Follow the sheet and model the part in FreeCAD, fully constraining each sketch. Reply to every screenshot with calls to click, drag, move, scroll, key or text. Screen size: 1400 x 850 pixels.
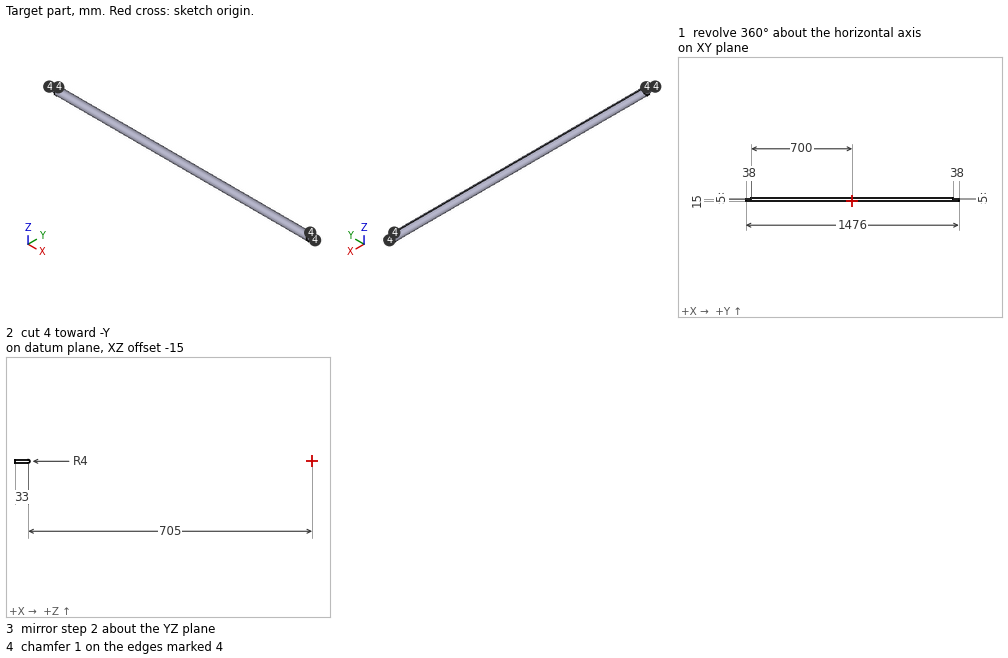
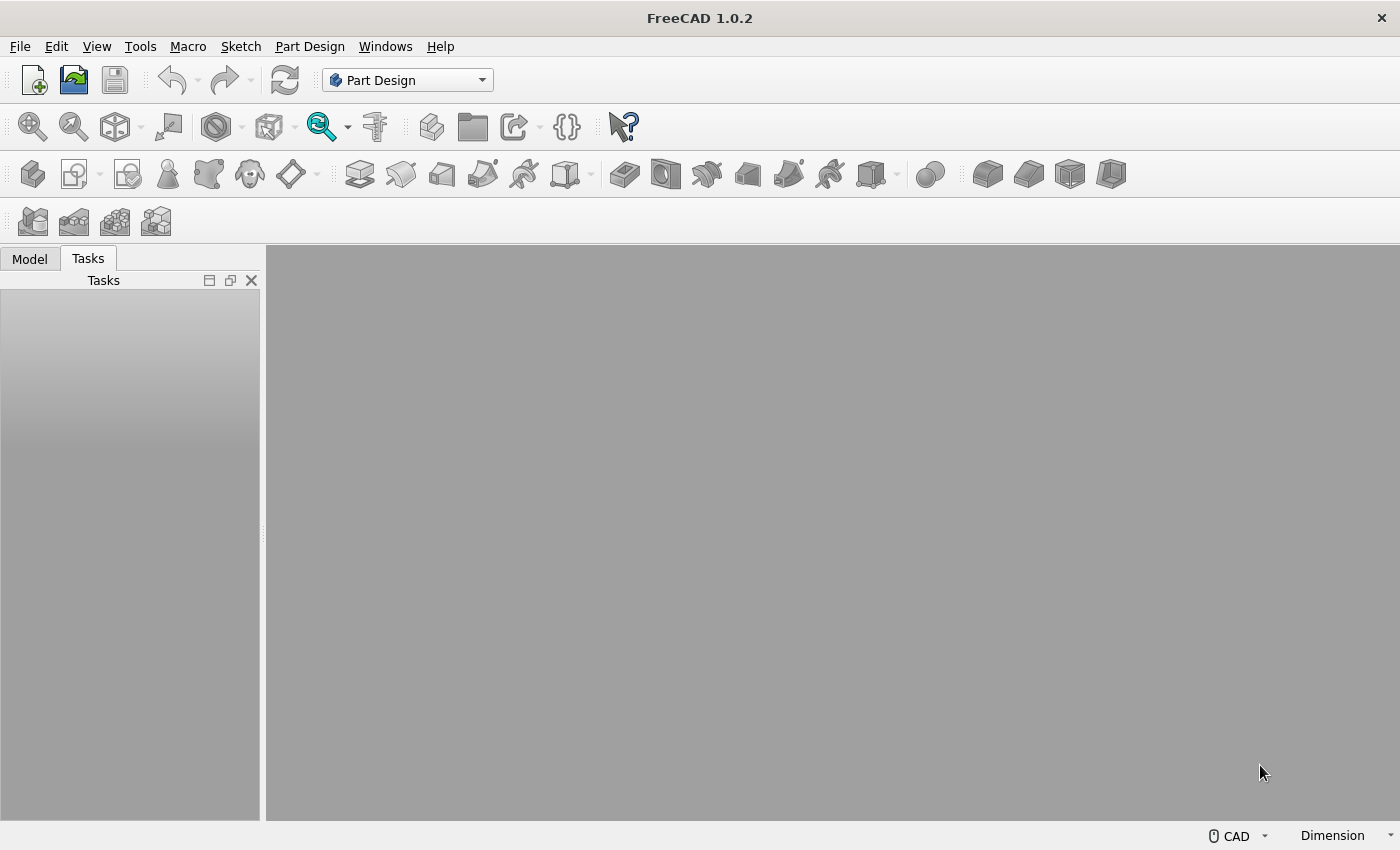
click(33, 80)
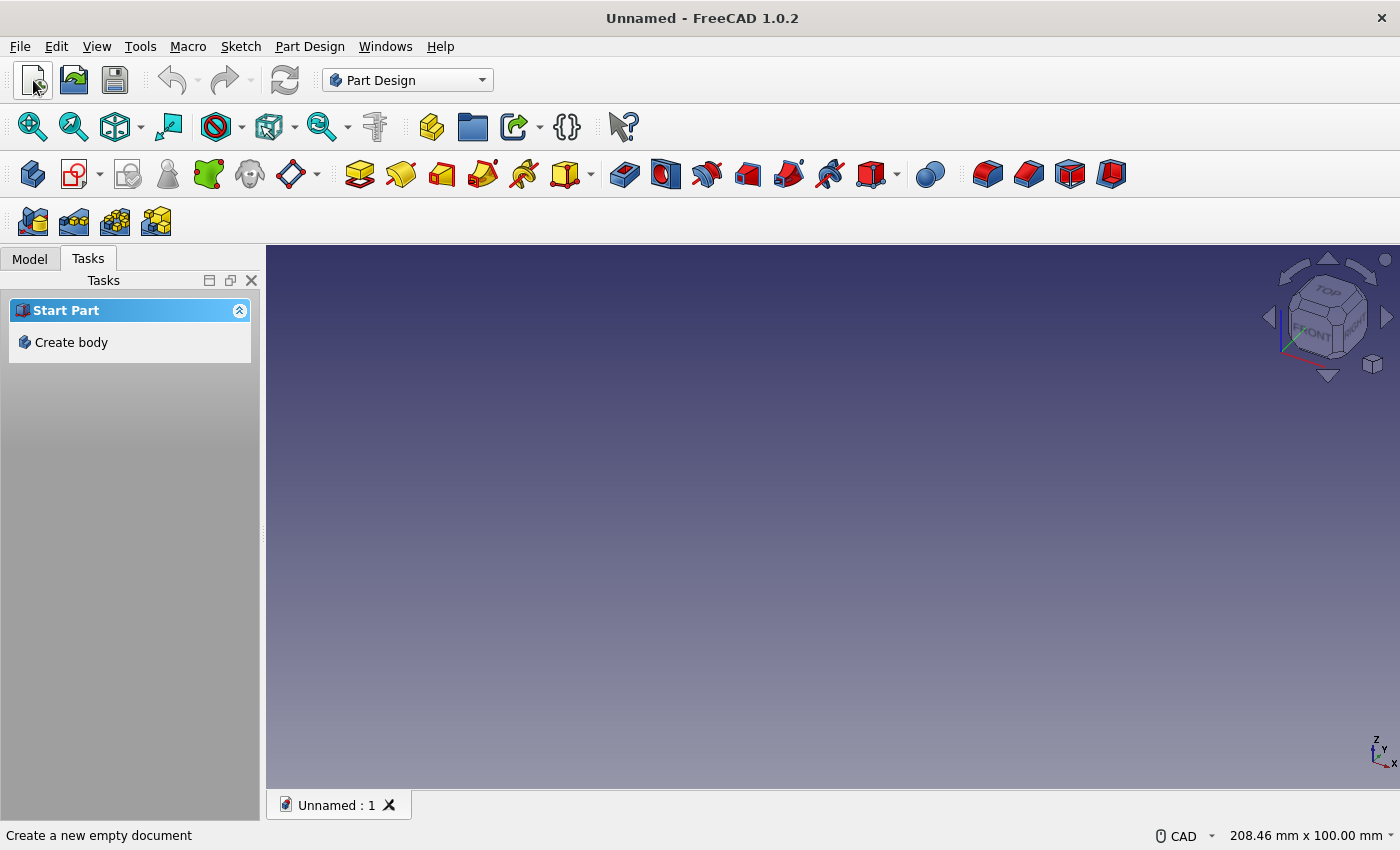
click(74, 174)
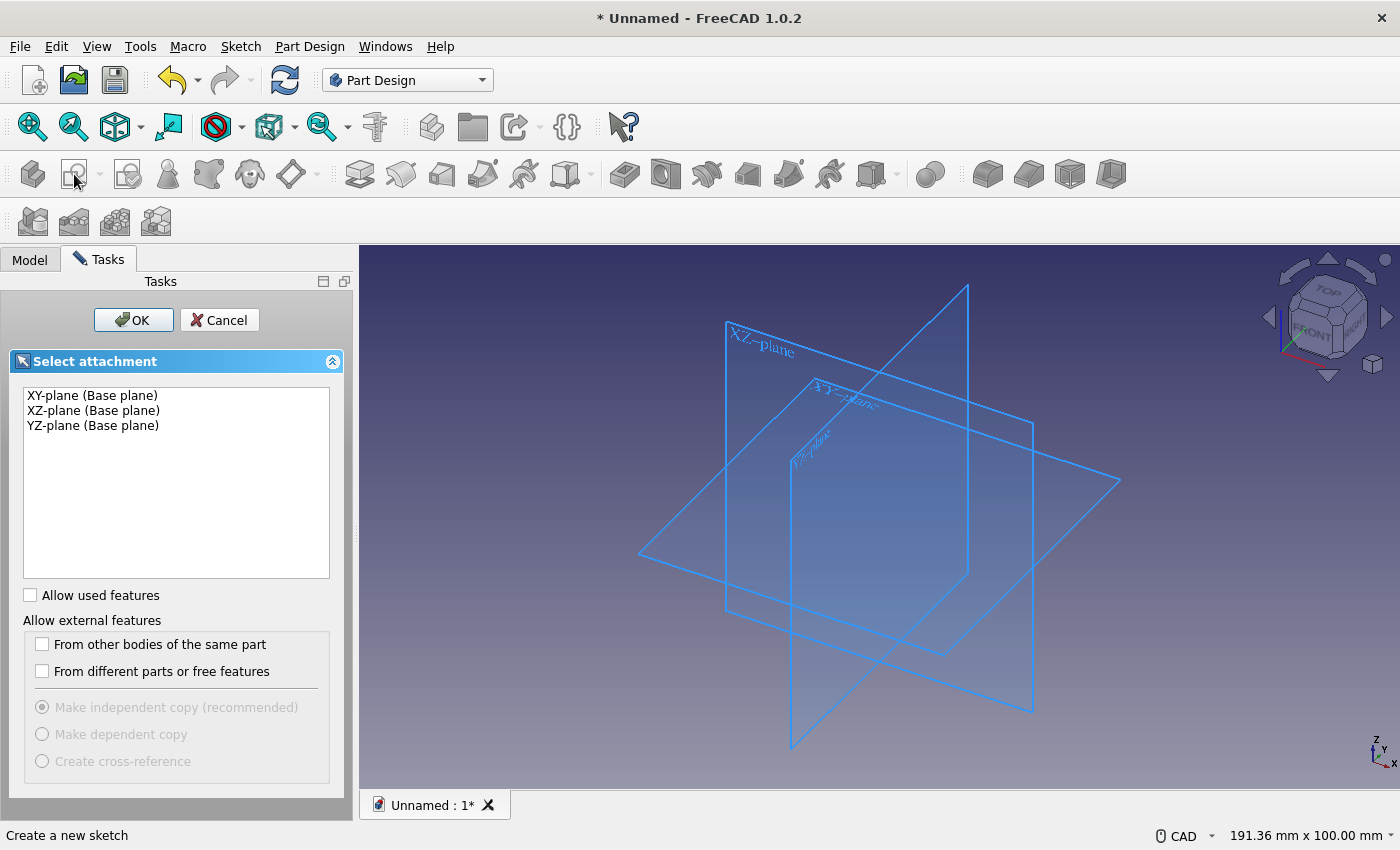
click(84, 396)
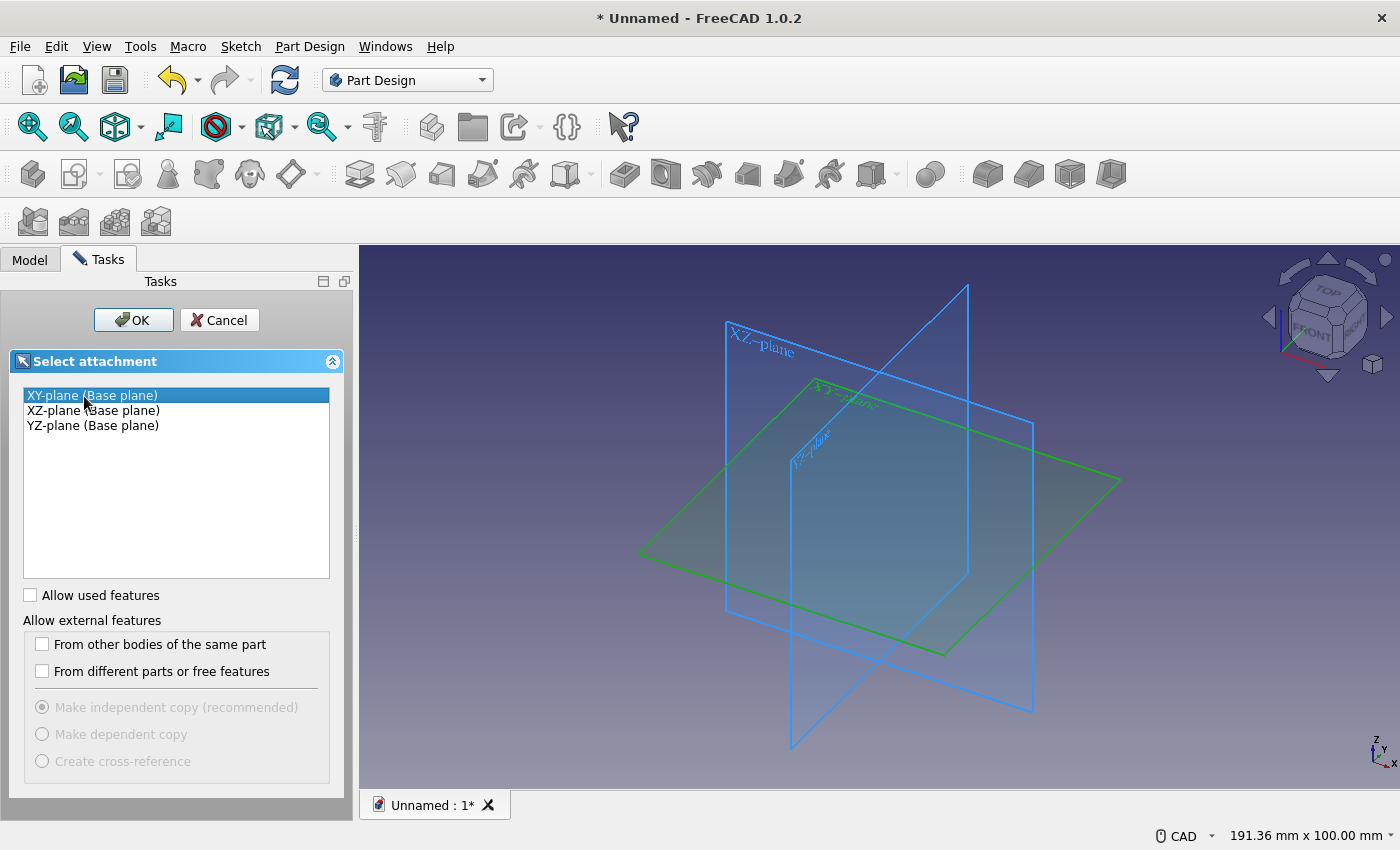
click(134, 320)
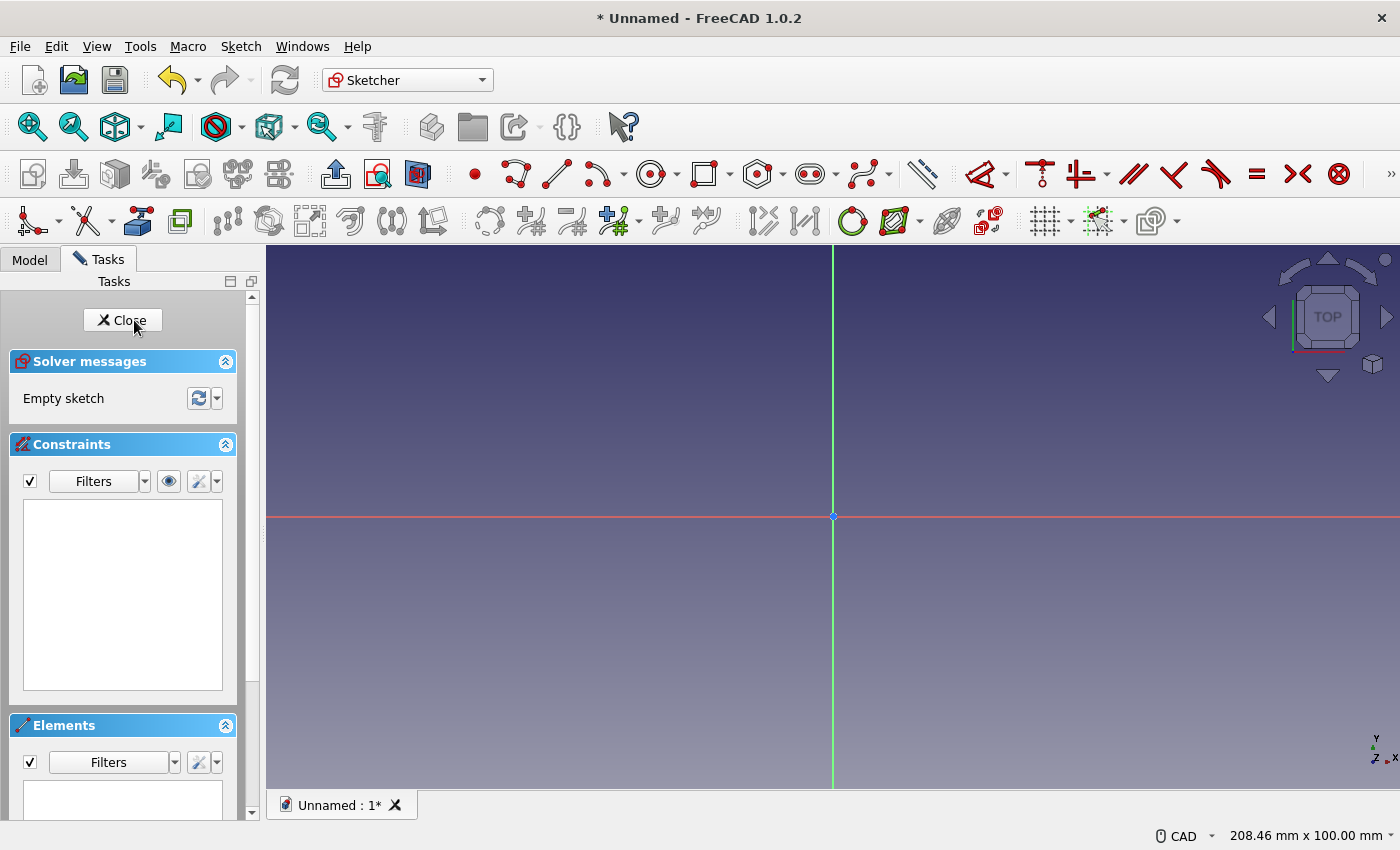
scroll(758, 522, down, 12)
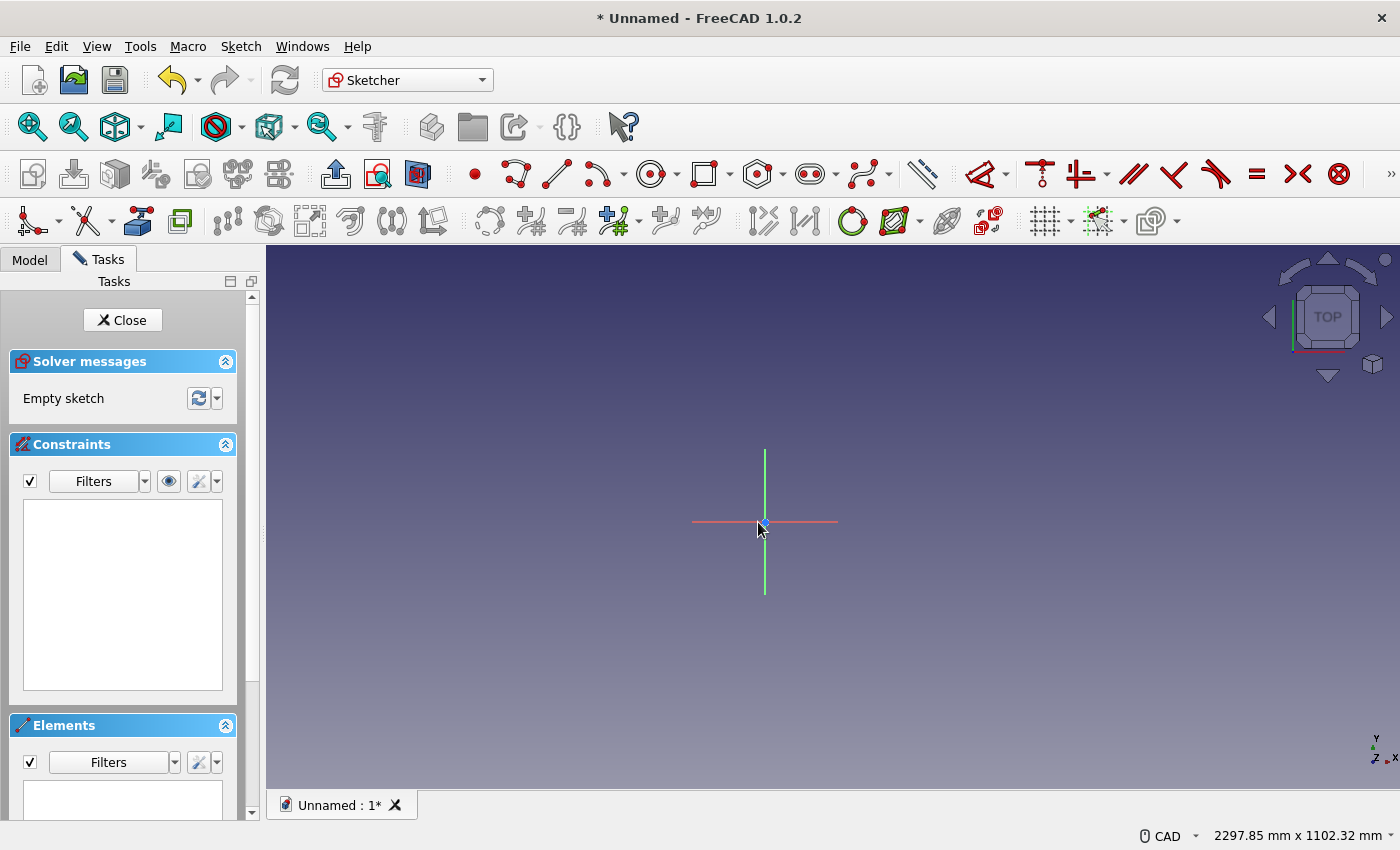
click(516, 174)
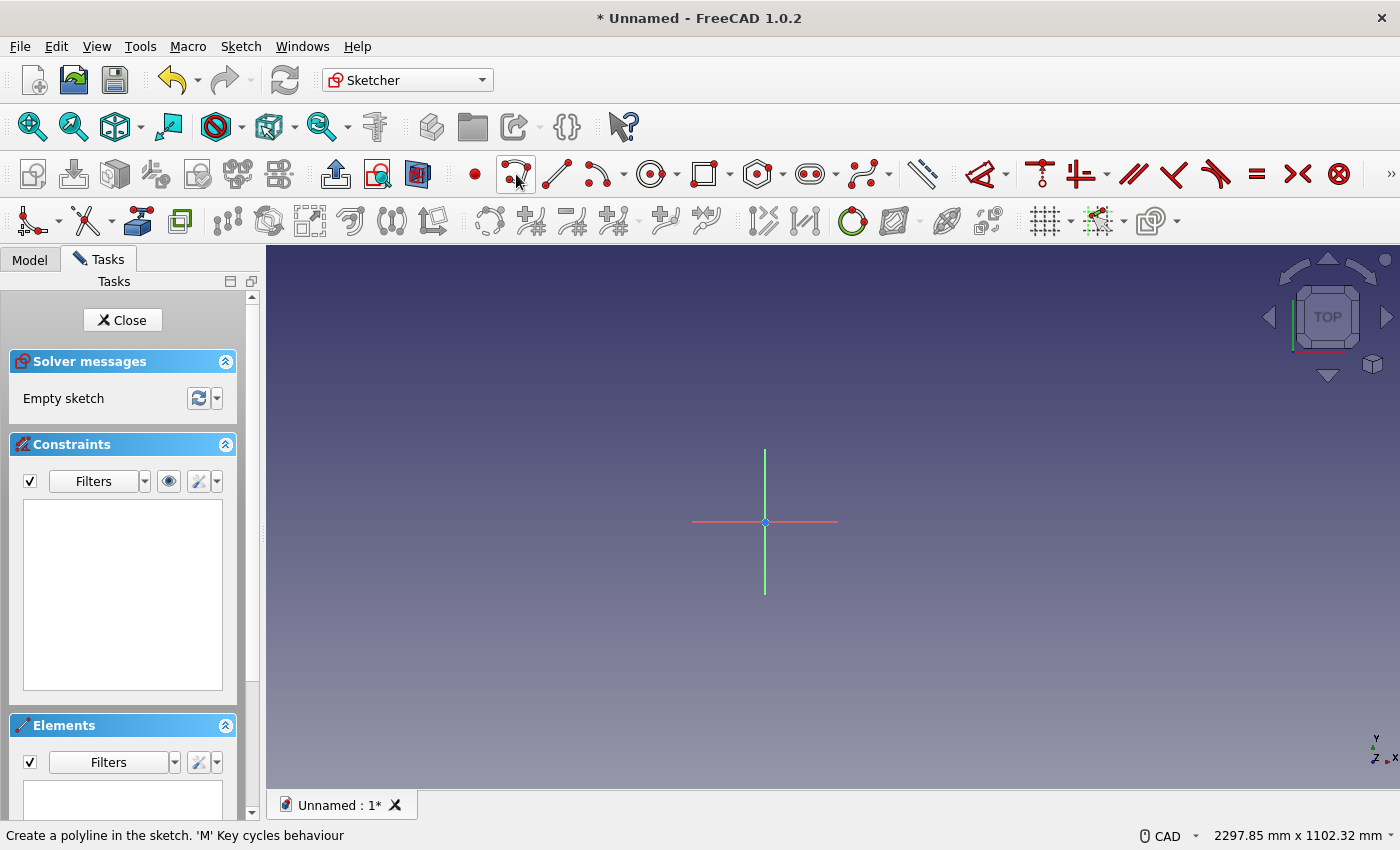
scroll(420, 515, up, 4)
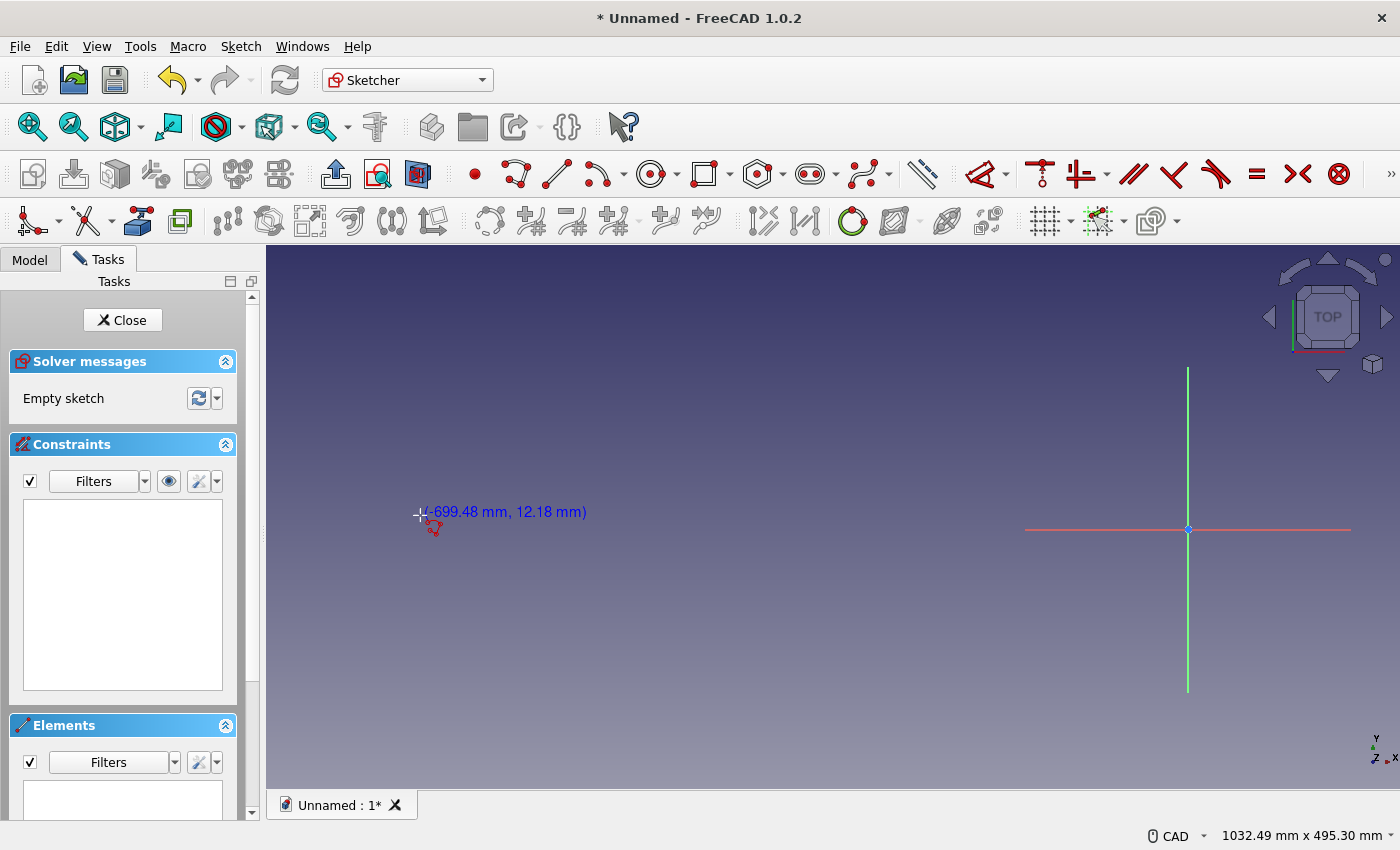
click(419, 514)
click(378, 514)
click(378, 530)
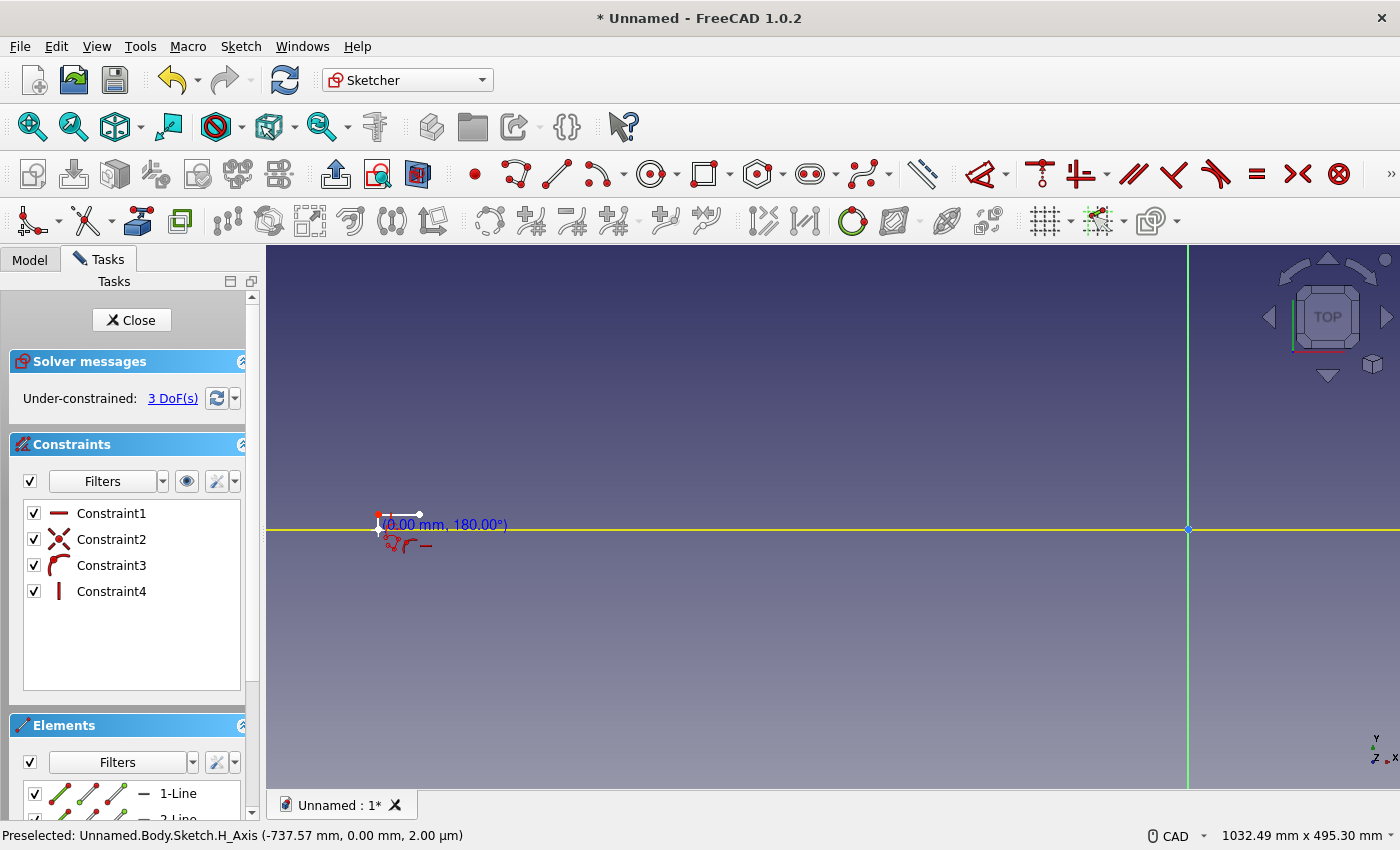
scroll(419, 515, down, 4)